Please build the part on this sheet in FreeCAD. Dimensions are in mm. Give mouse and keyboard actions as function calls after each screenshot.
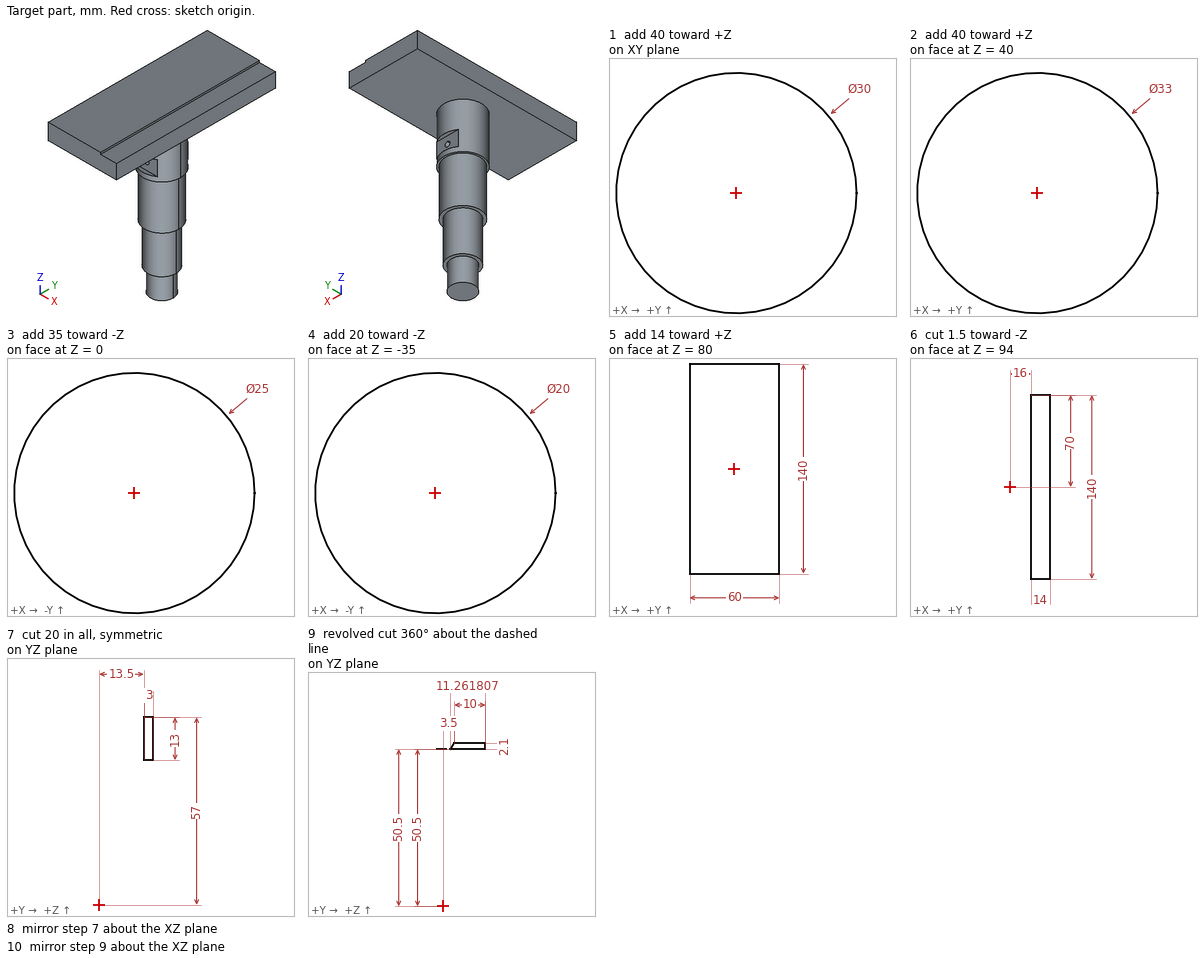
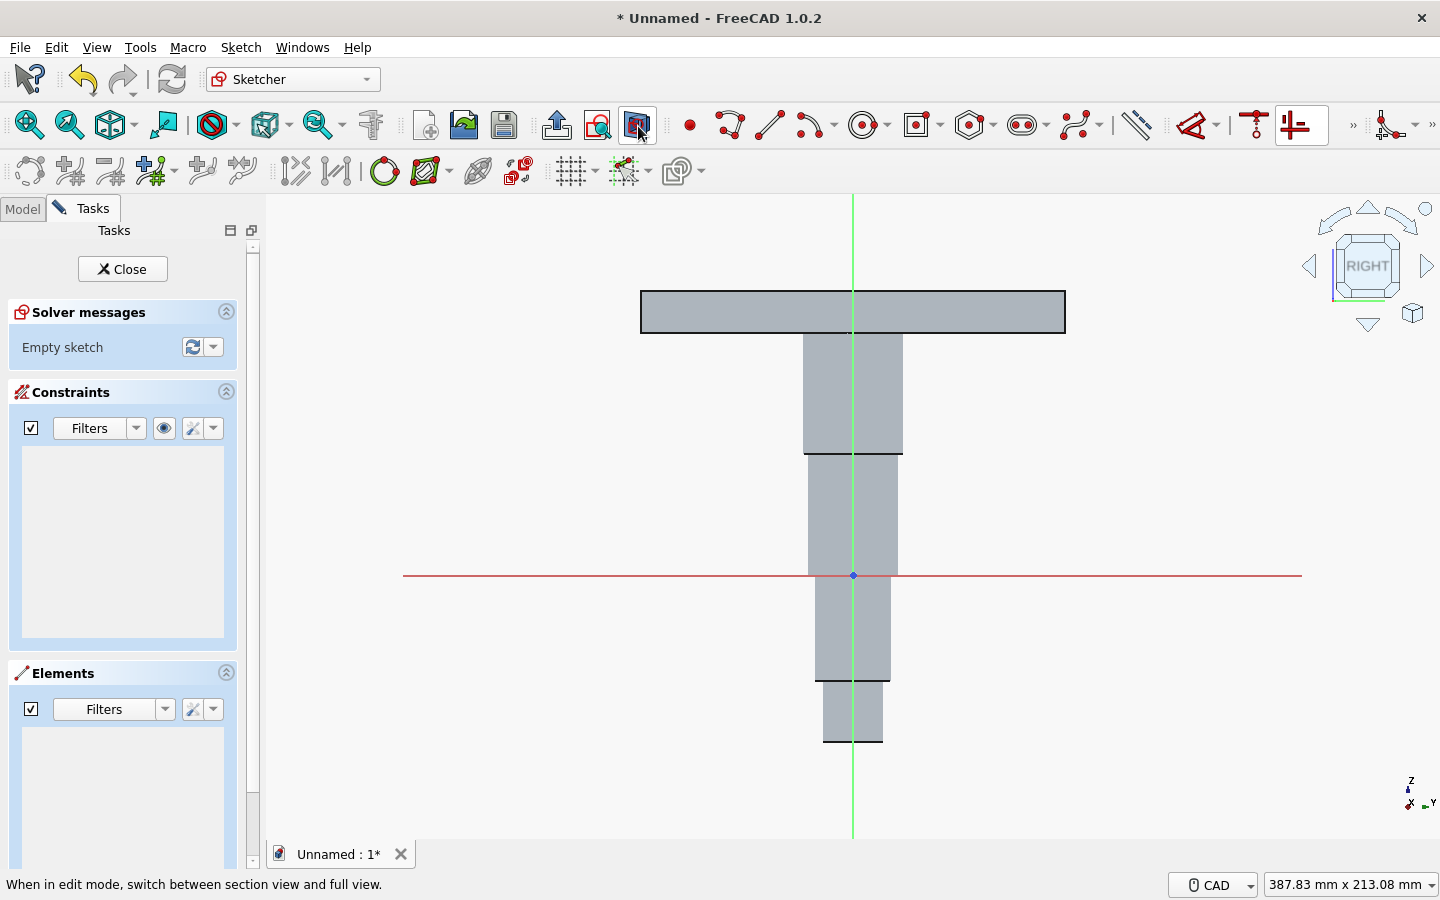
scroll(910, 413, up, 12)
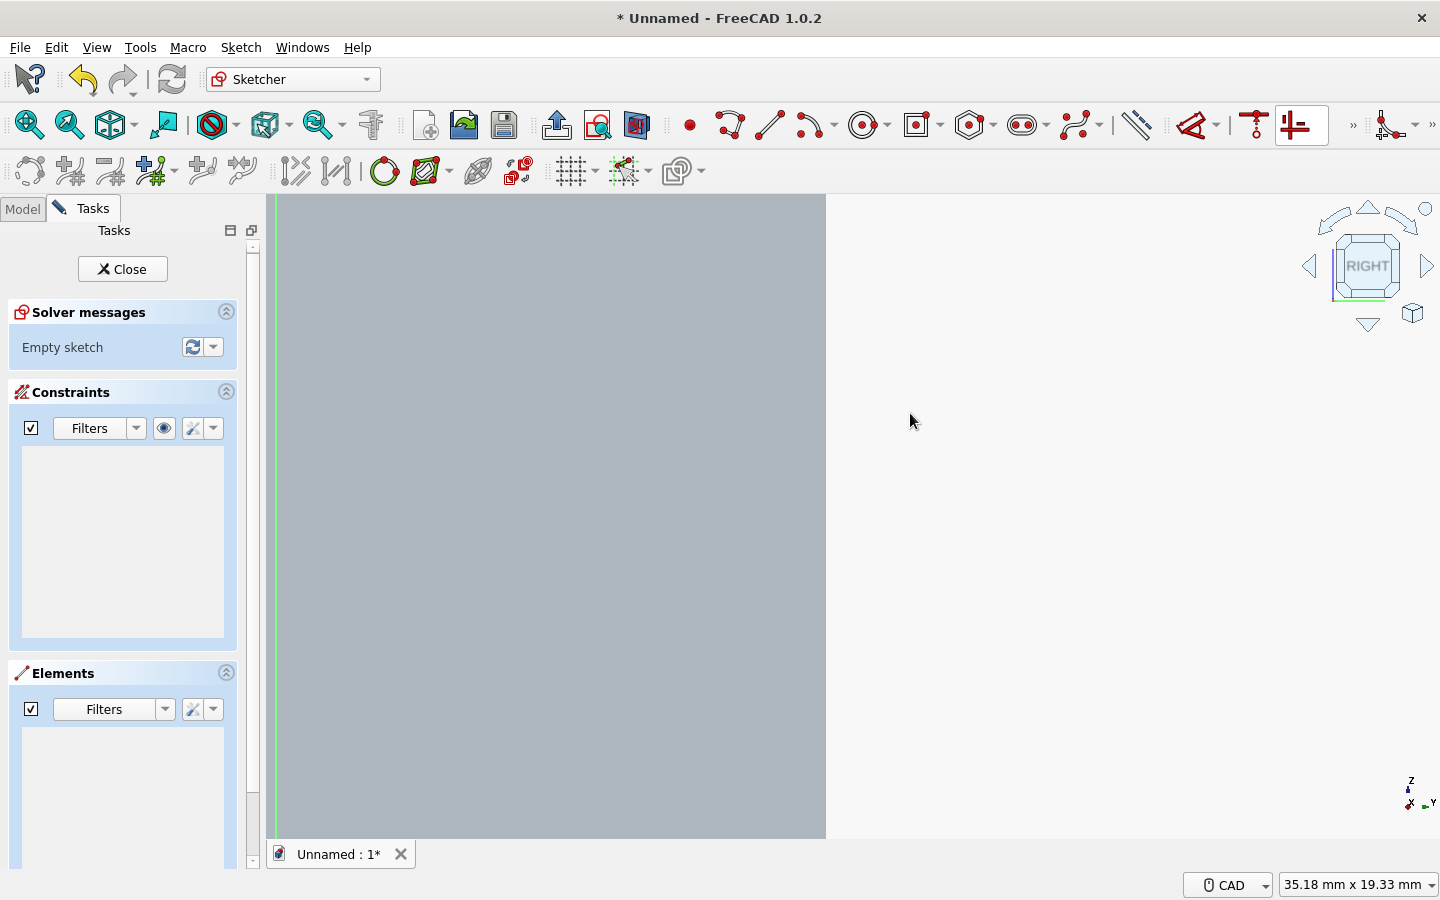
key(g)
key(r)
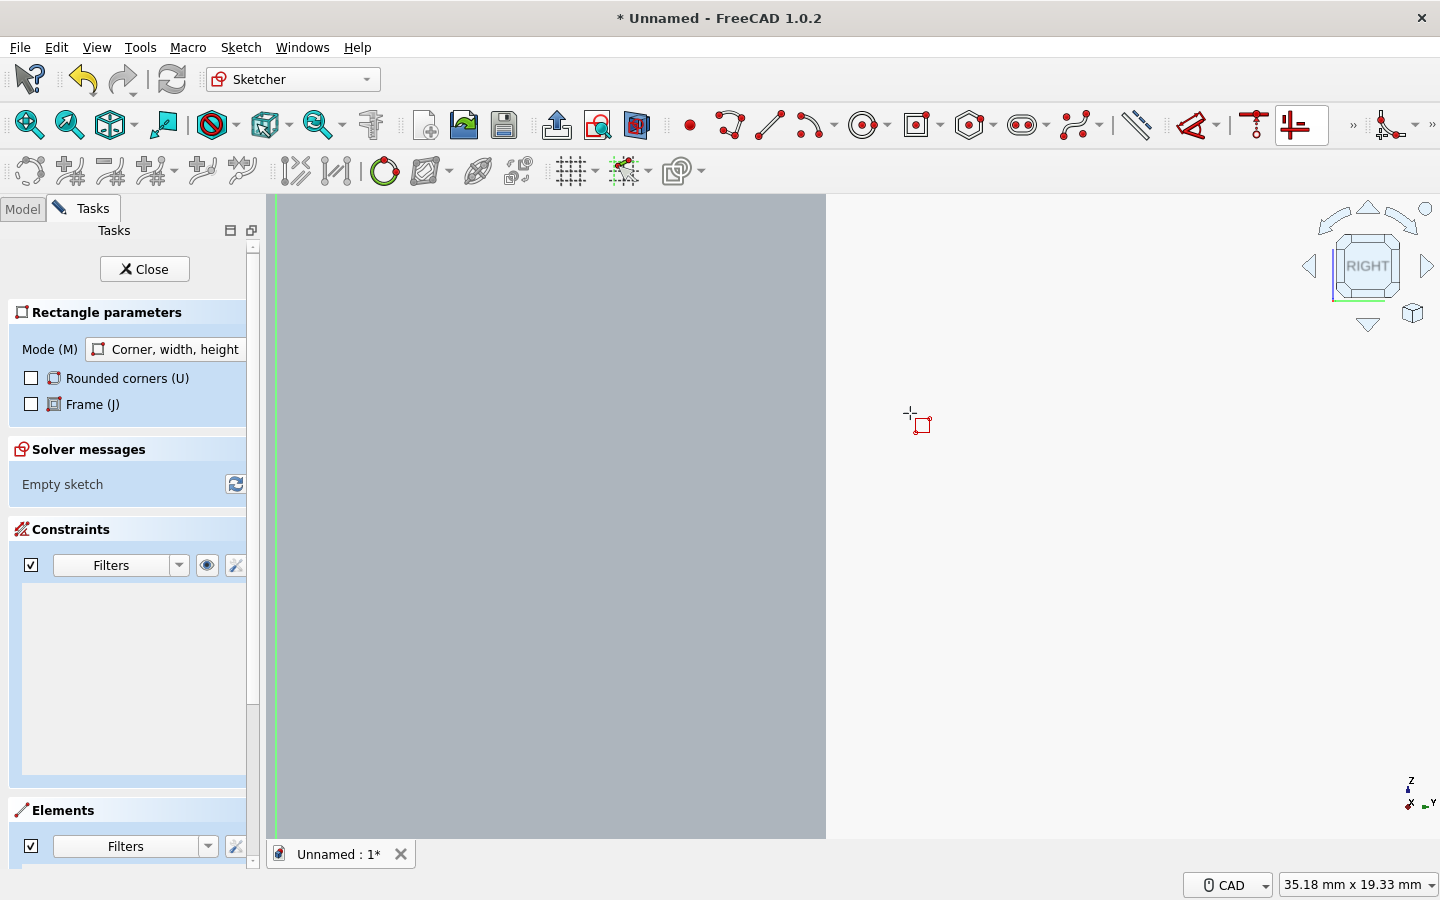
click(727, 299)
move(827, 733)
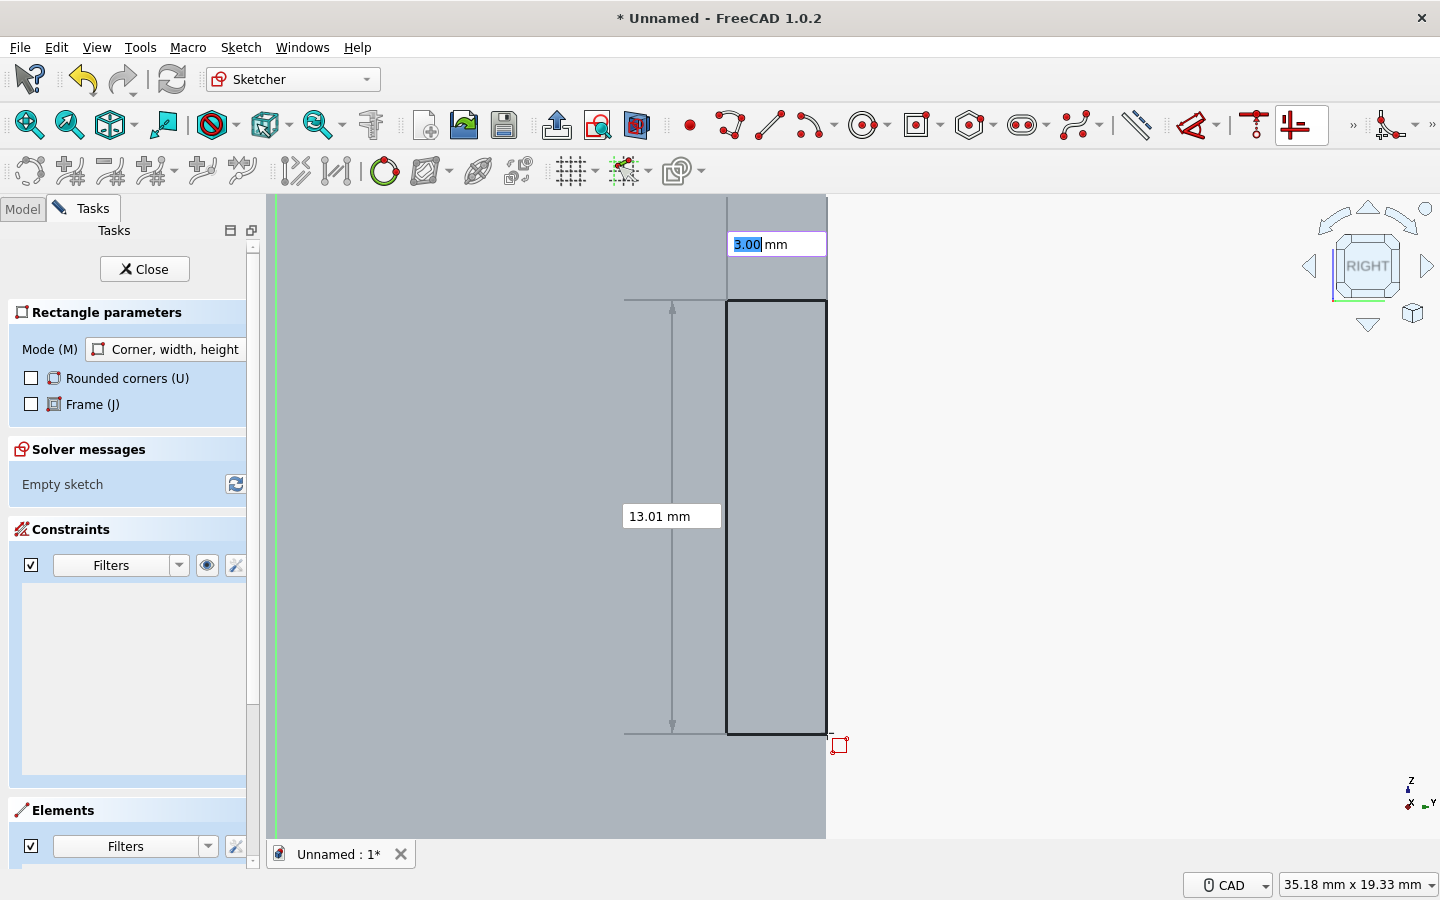
text(3)
key(Tab)
text(13)
key(Return)
key(Escape)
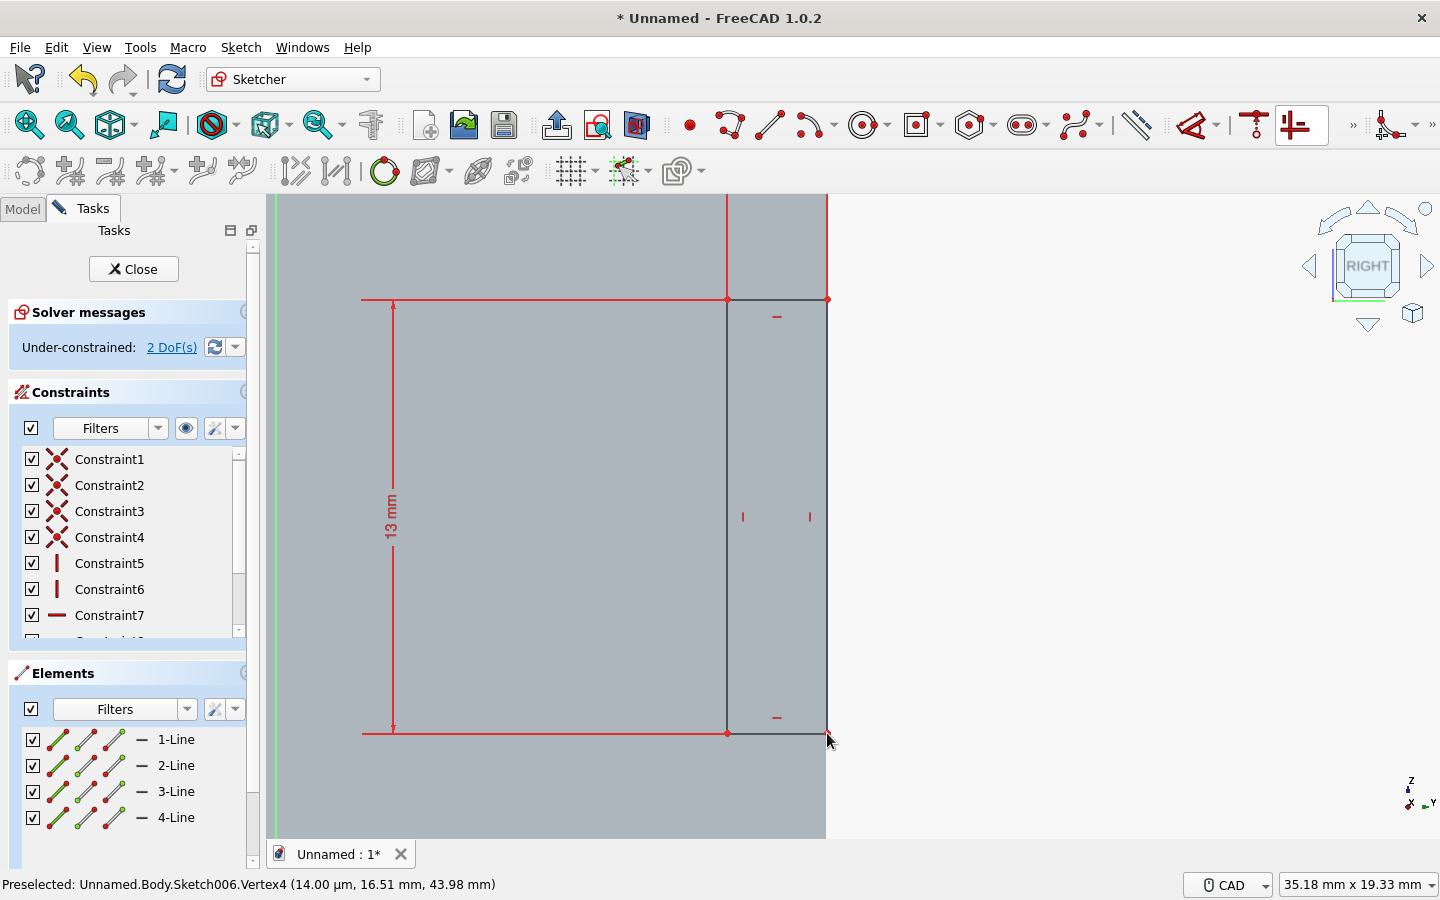
click(1192, 126)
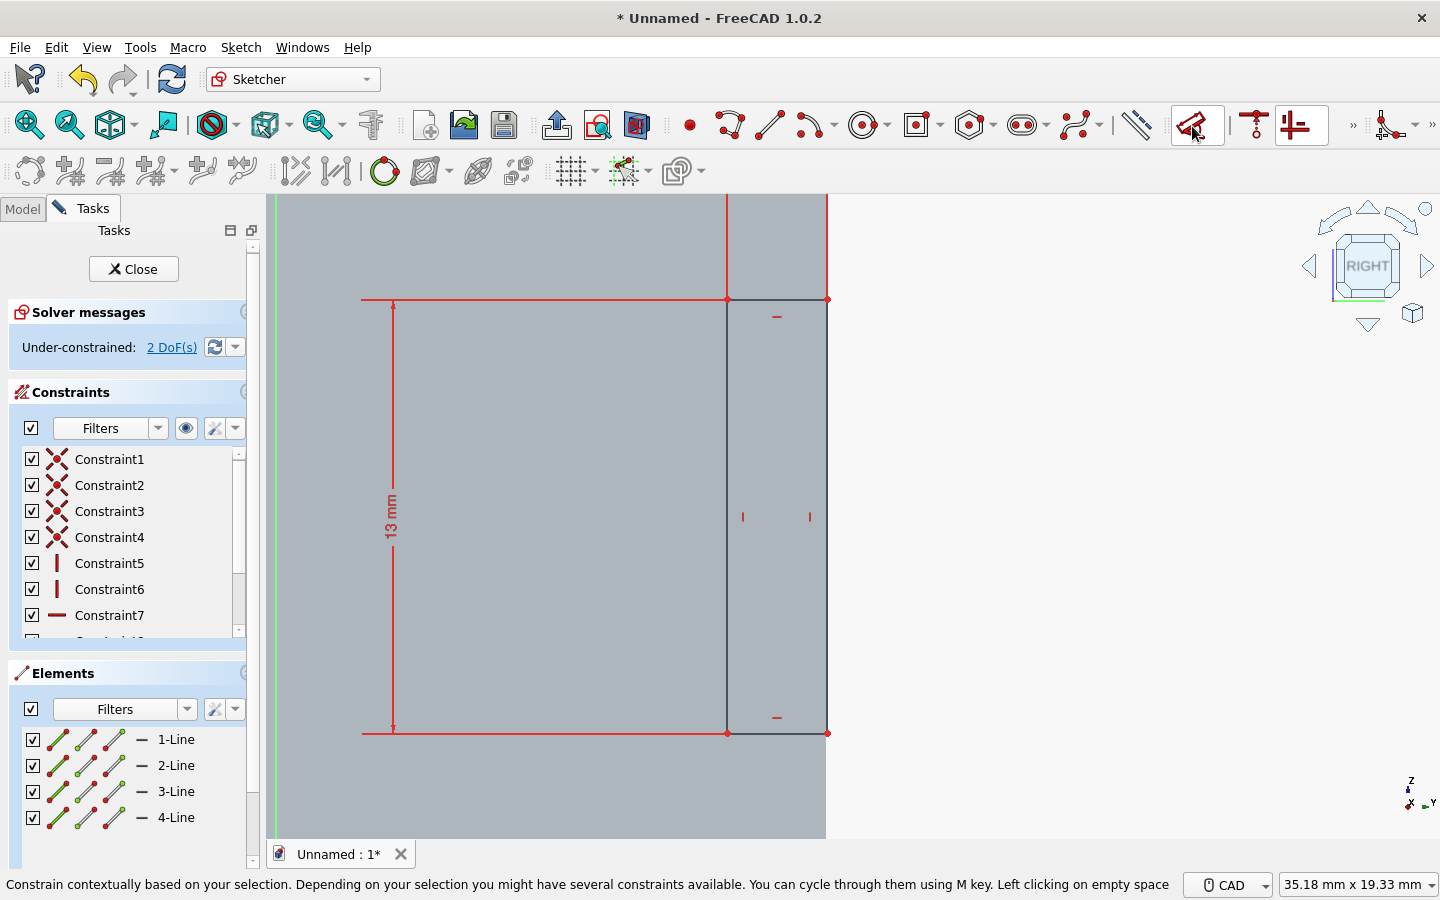
click(727, 300)
click(761, 555)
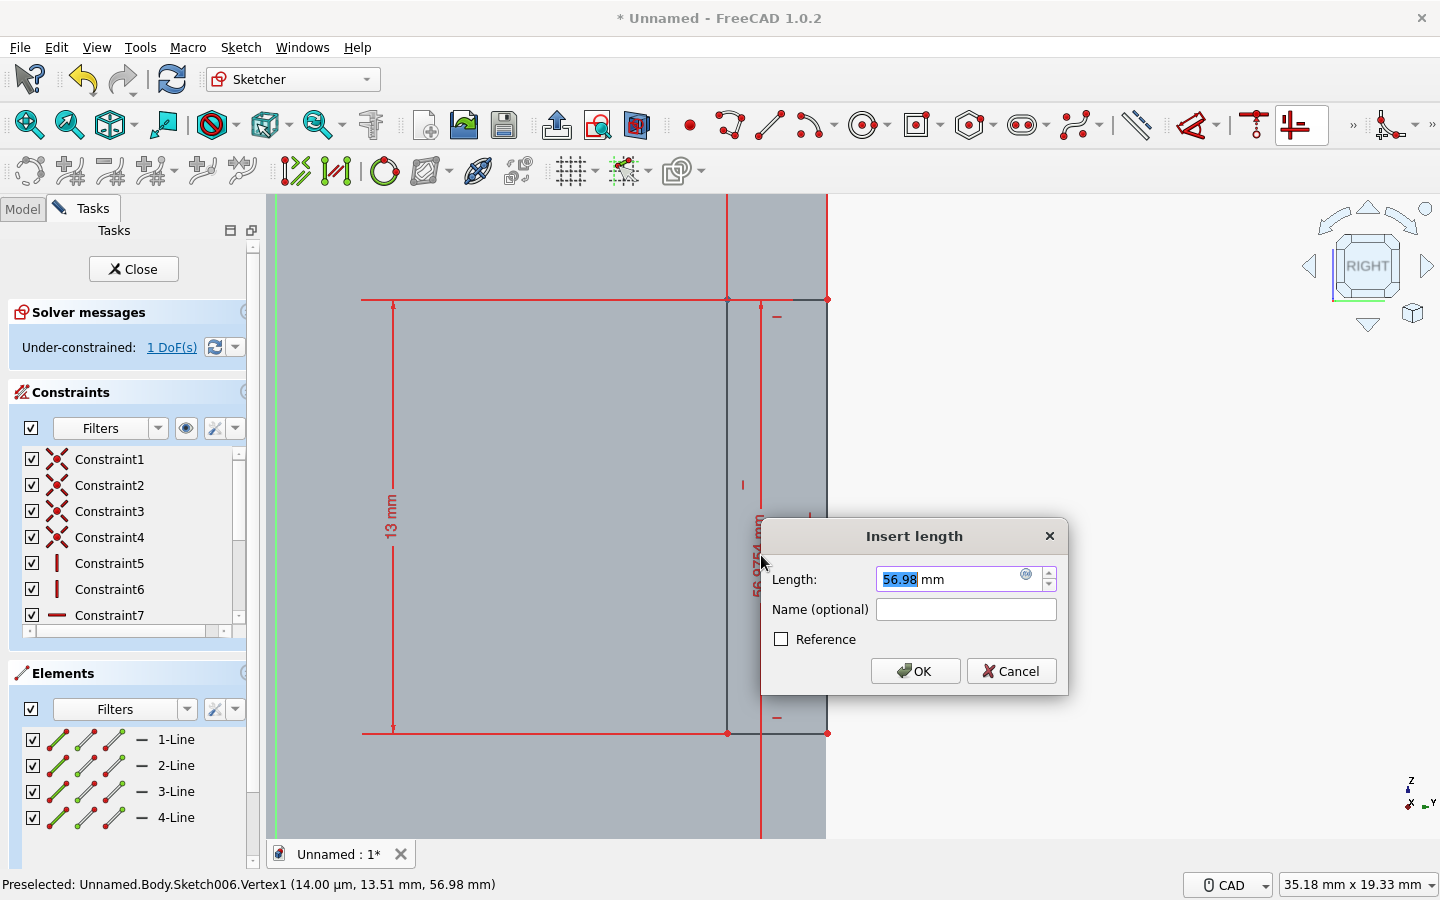
text(57)
key(Return)